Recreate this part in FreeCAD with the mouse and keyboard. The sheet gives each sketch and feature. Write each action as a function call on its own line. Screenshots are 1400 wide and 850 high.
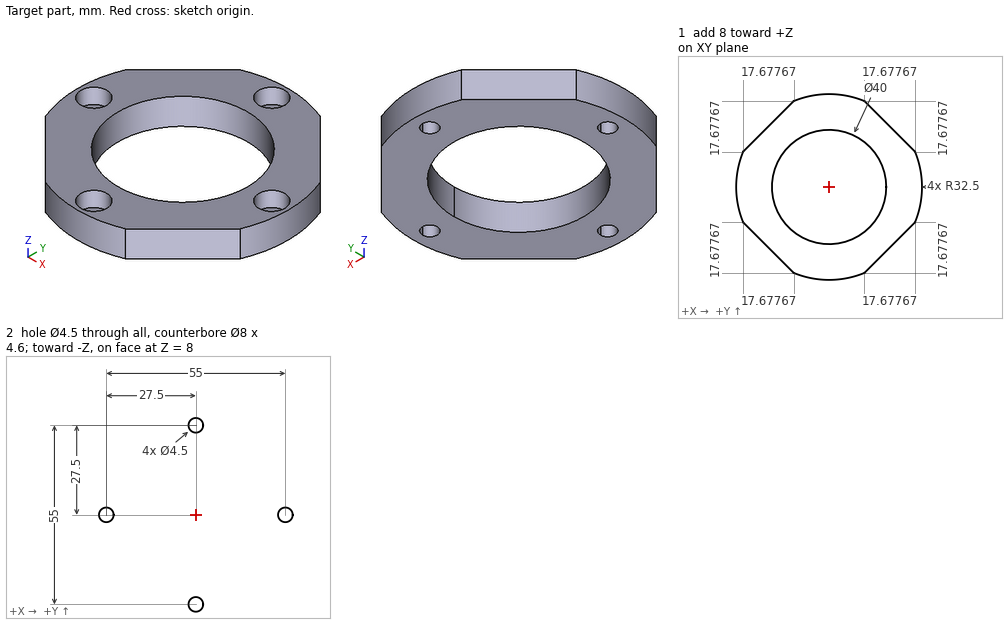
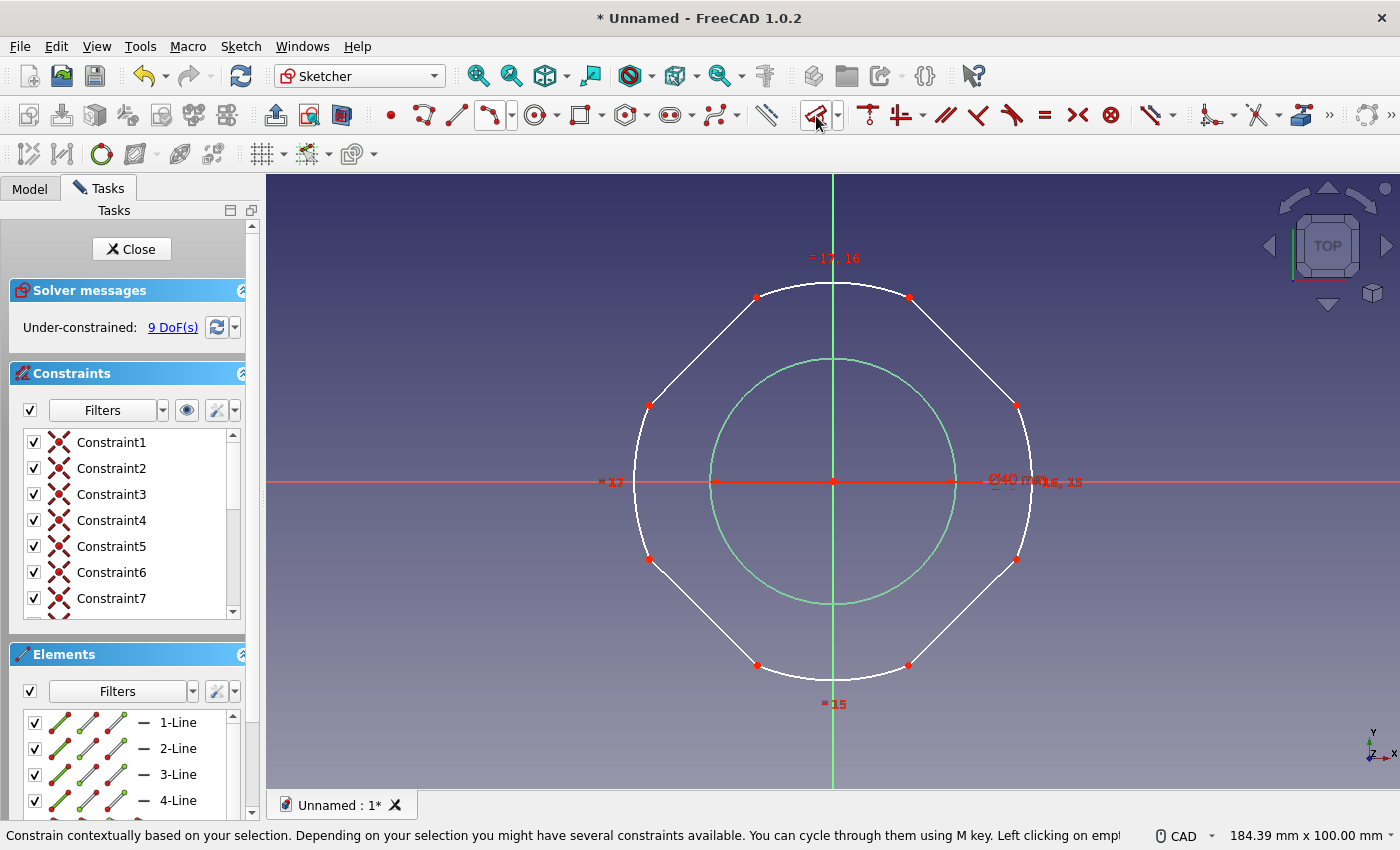
click(802, 678)
click(797, 710)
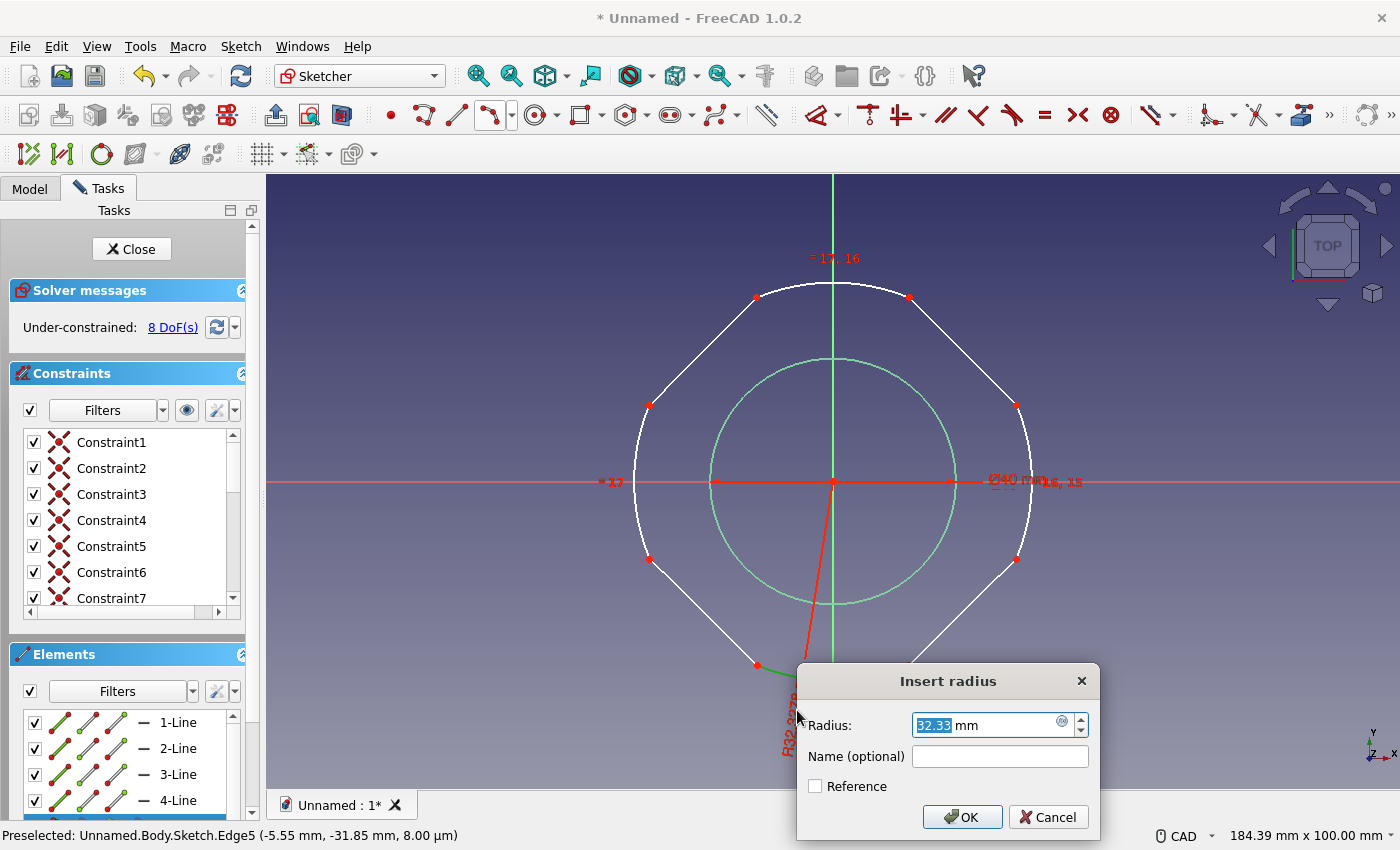
text(32.5)
key(Return)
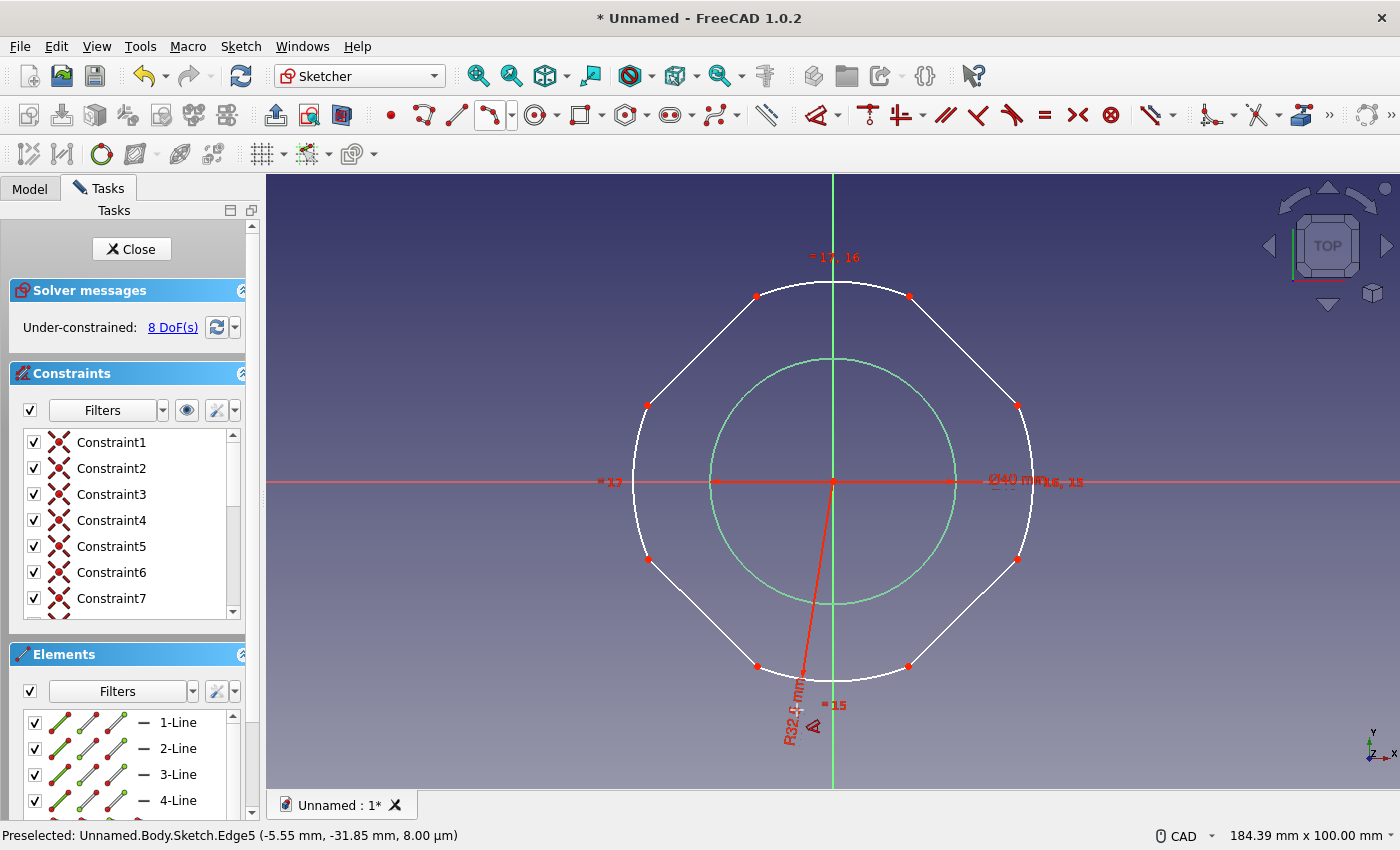
click(681, 591)
click(703, 700)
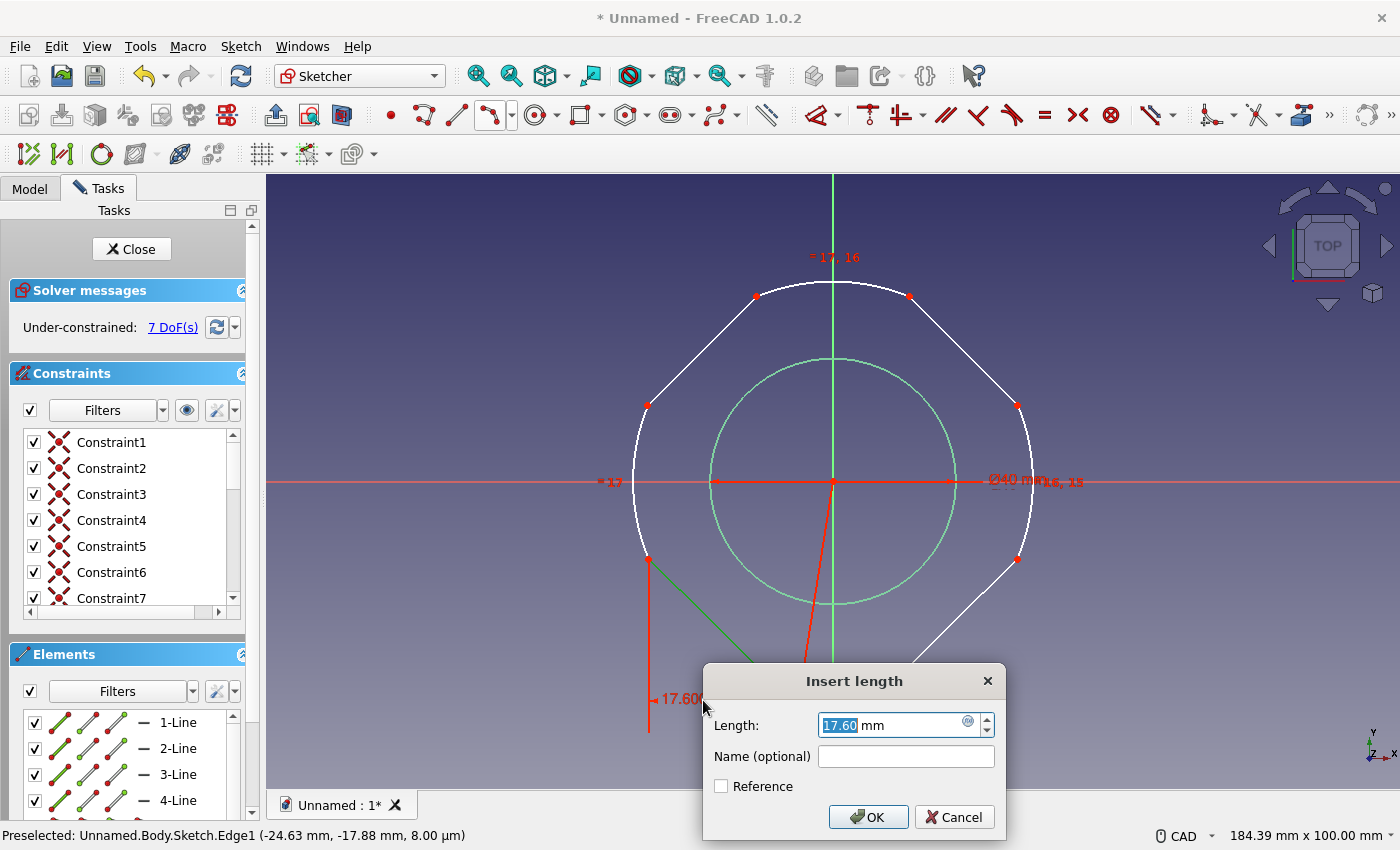
text(17.67767)
key(Return)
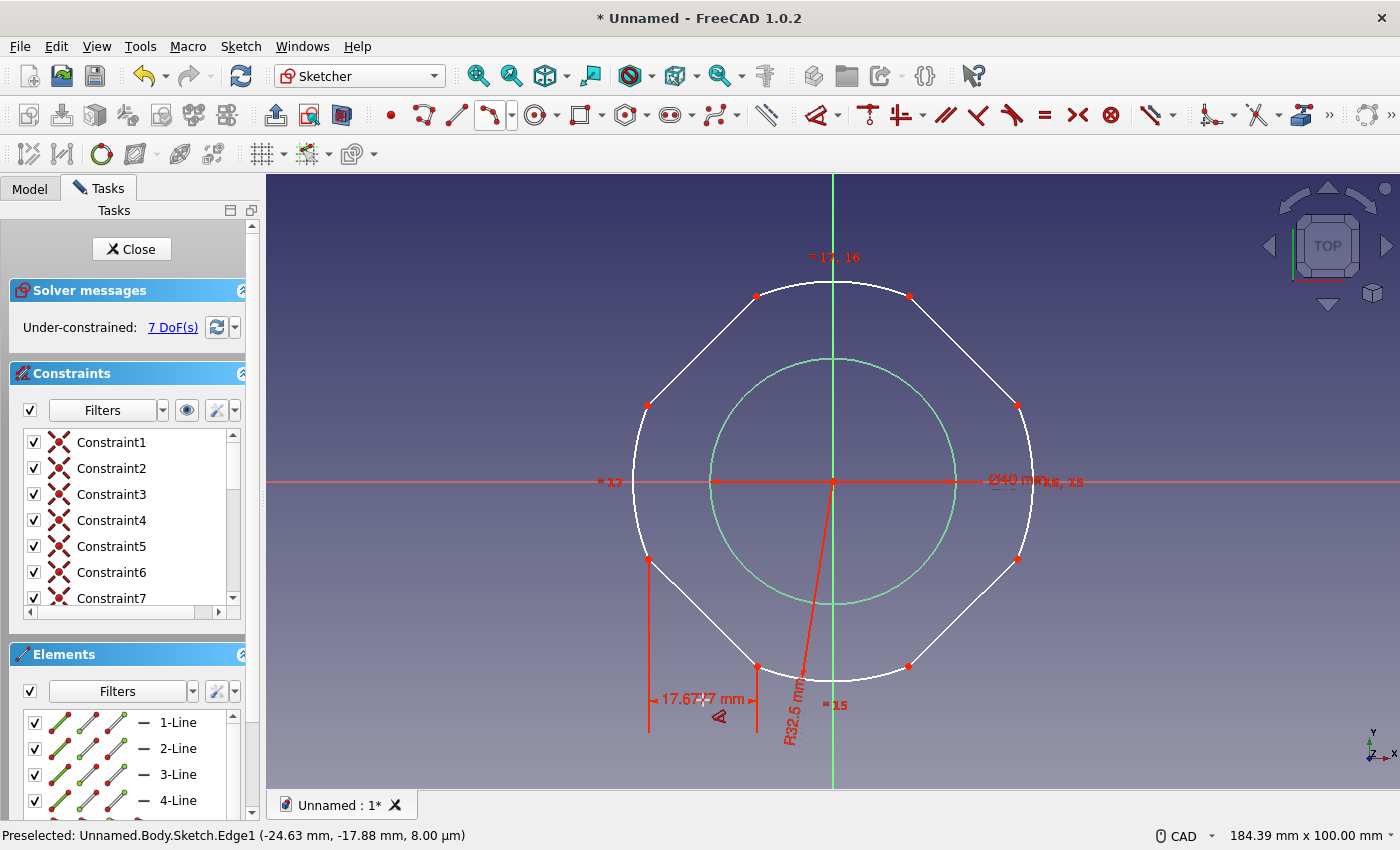
click(681, 591)
click(615, 613)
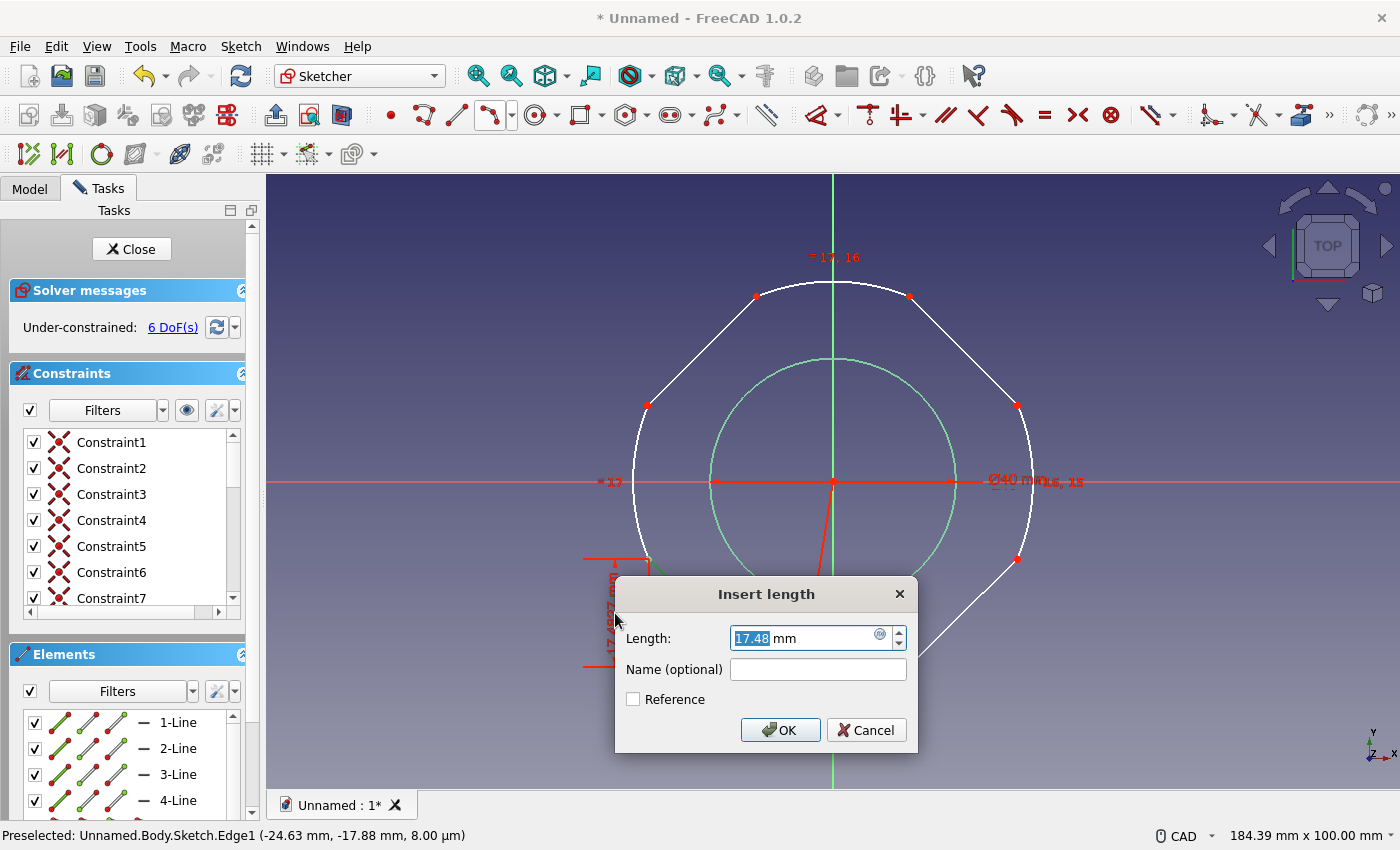
text(17.67767)
key(Return)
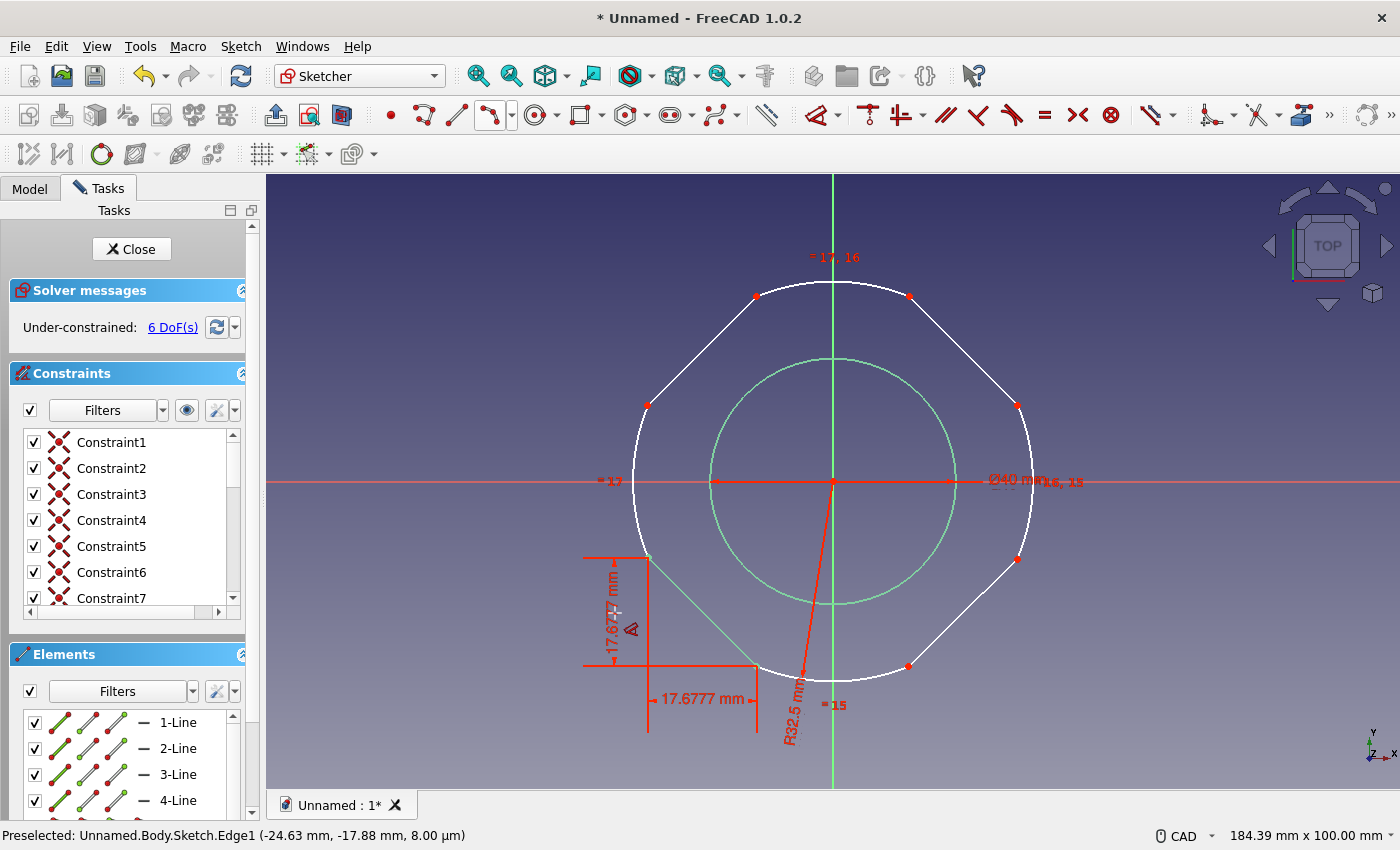
click(941, 634)
click(963, 700)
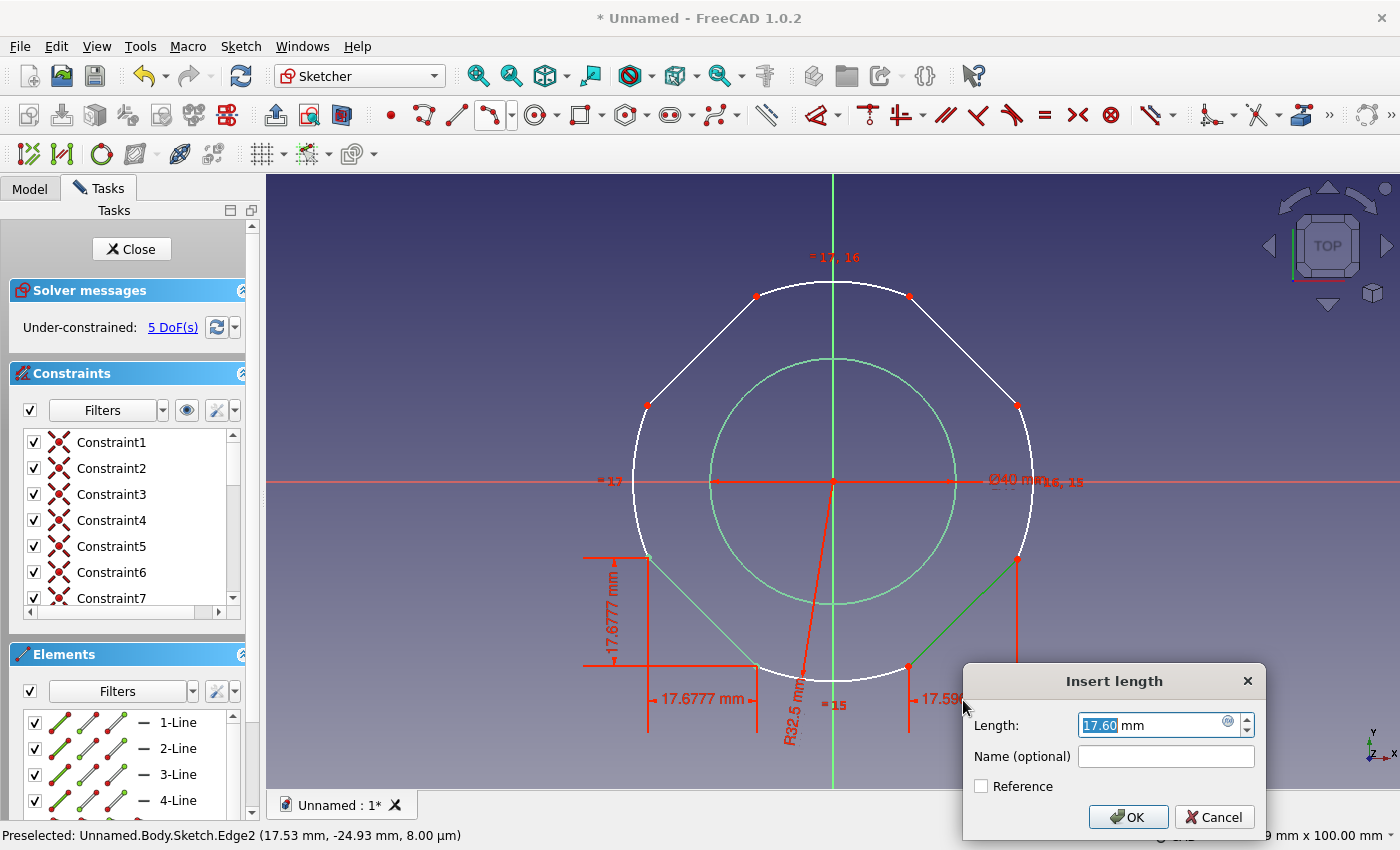
text(17.67767)
key(Return)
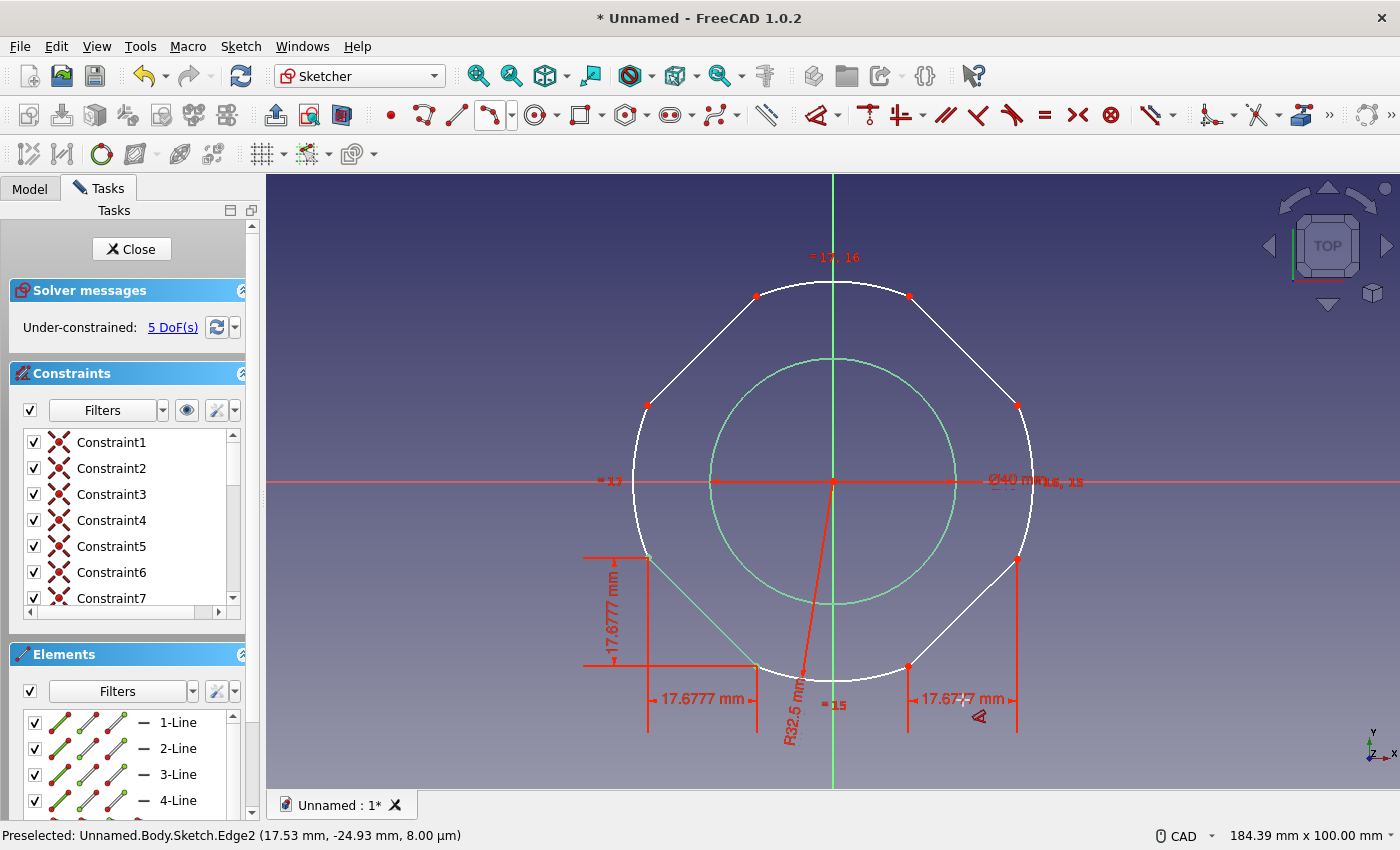
click(941, 634)
click(1051, 613)